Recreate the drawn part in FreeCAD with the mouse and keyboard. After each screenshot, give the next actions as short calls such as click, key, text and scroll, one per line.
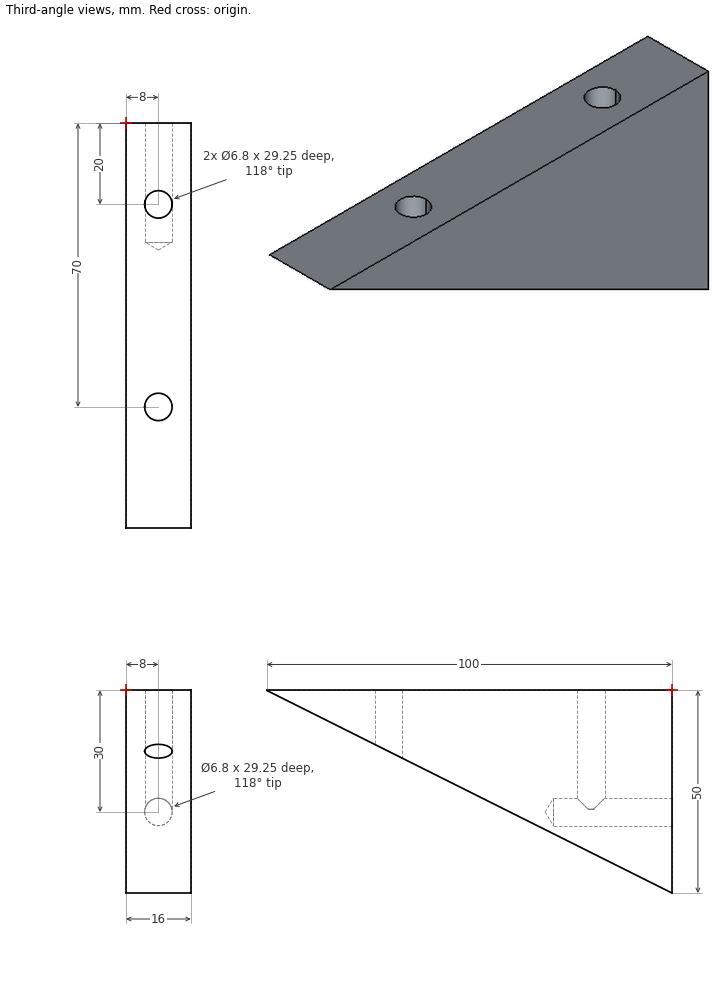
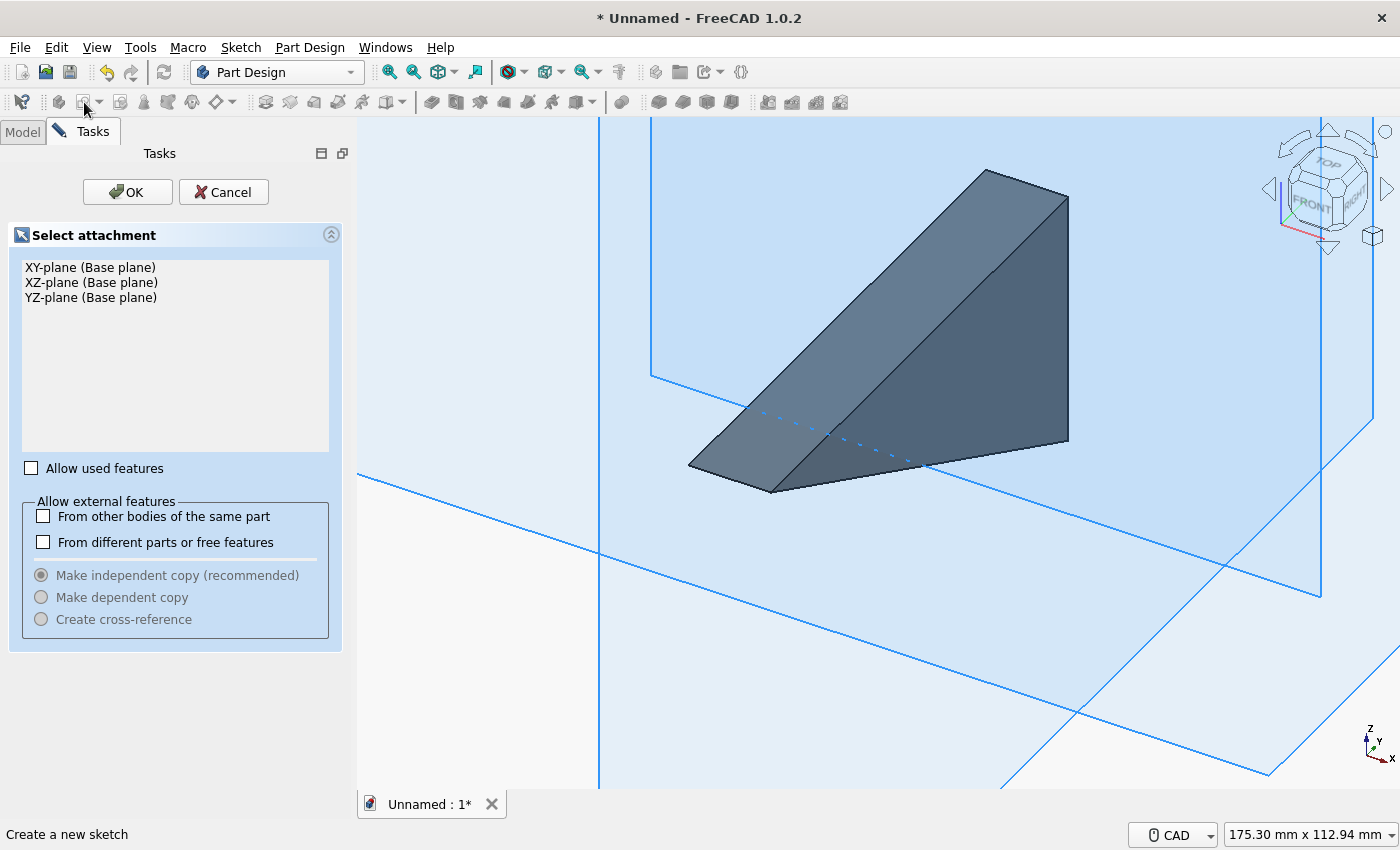
click(82, 282)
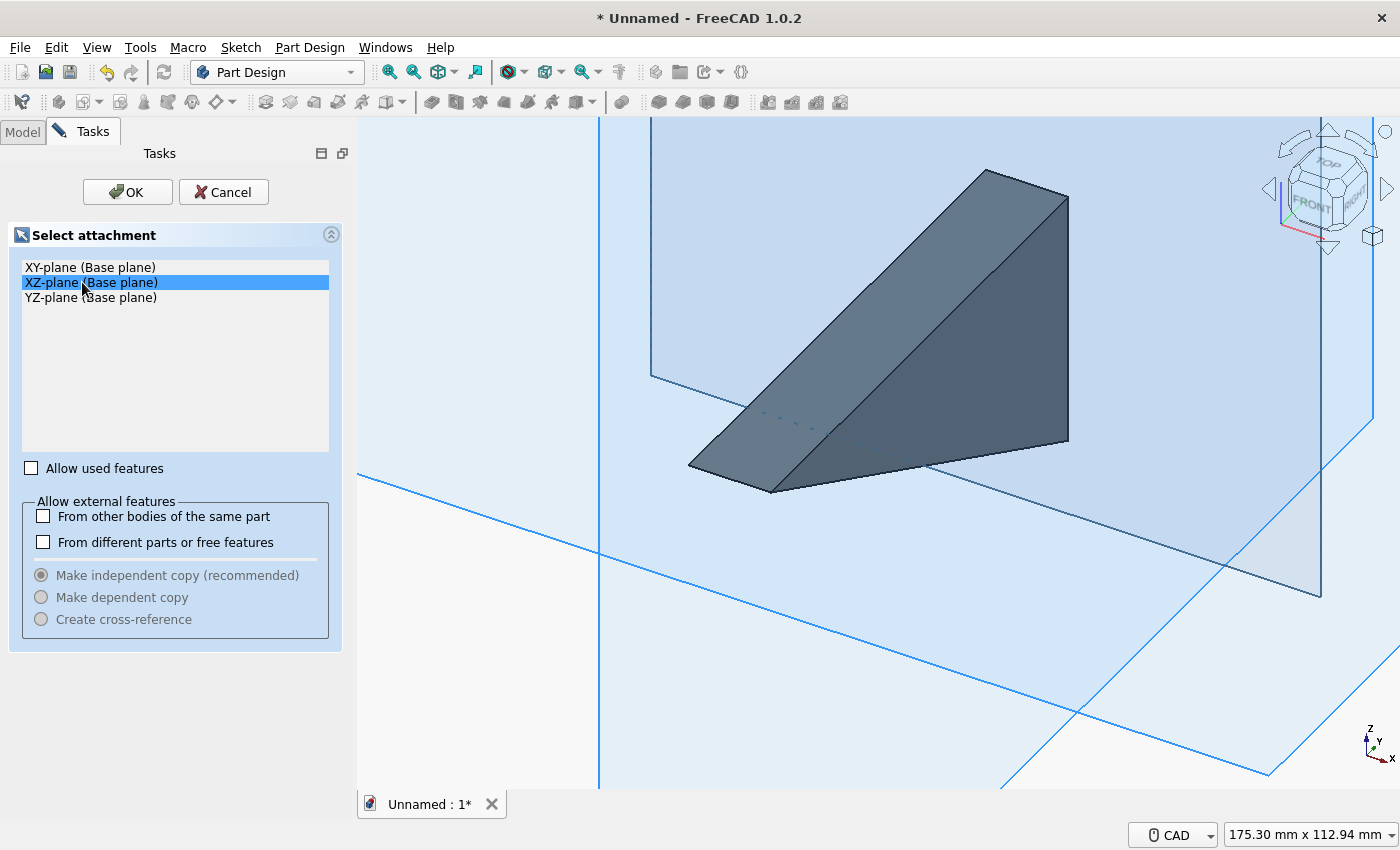
click(128, 192)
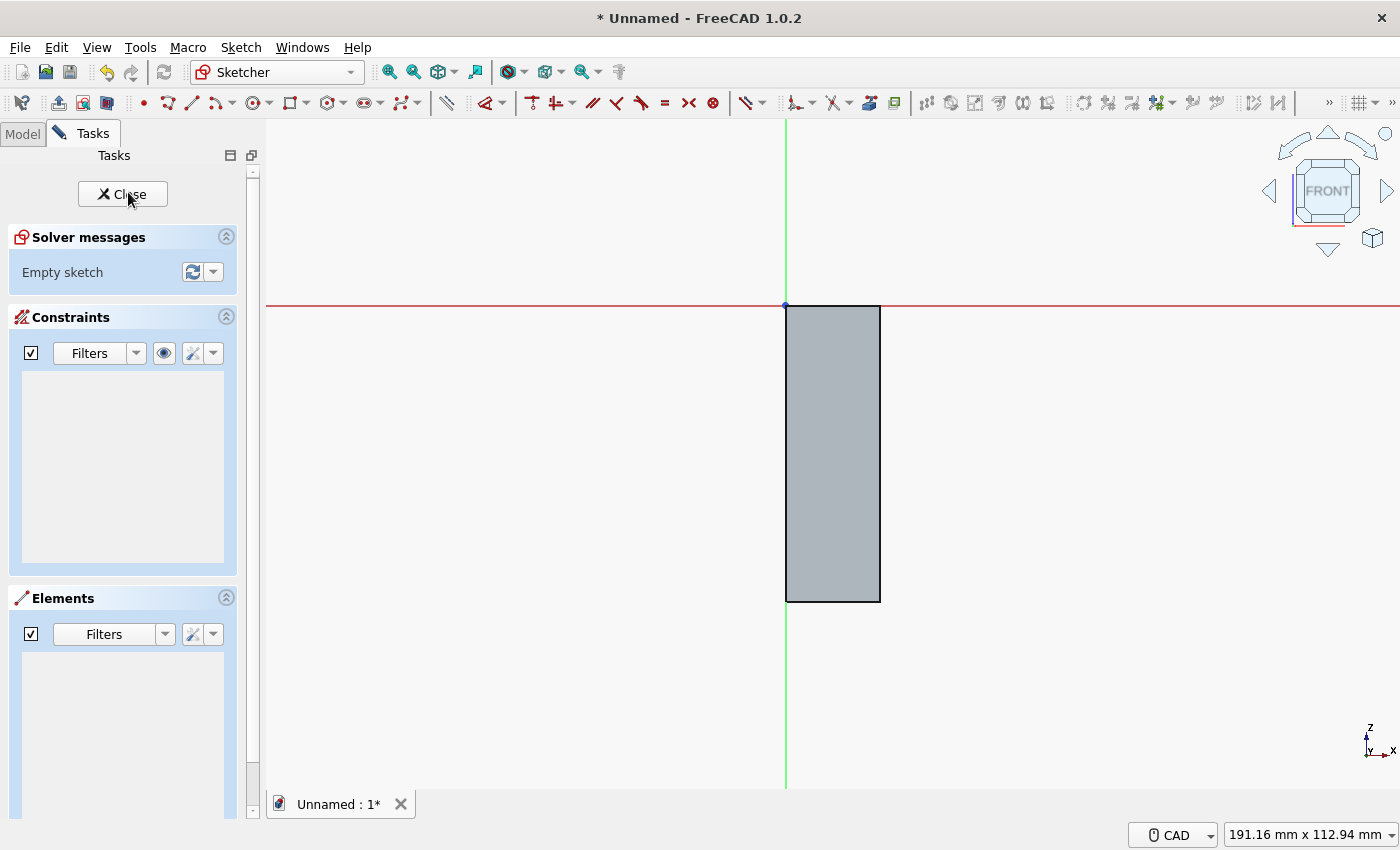
click(108, 104)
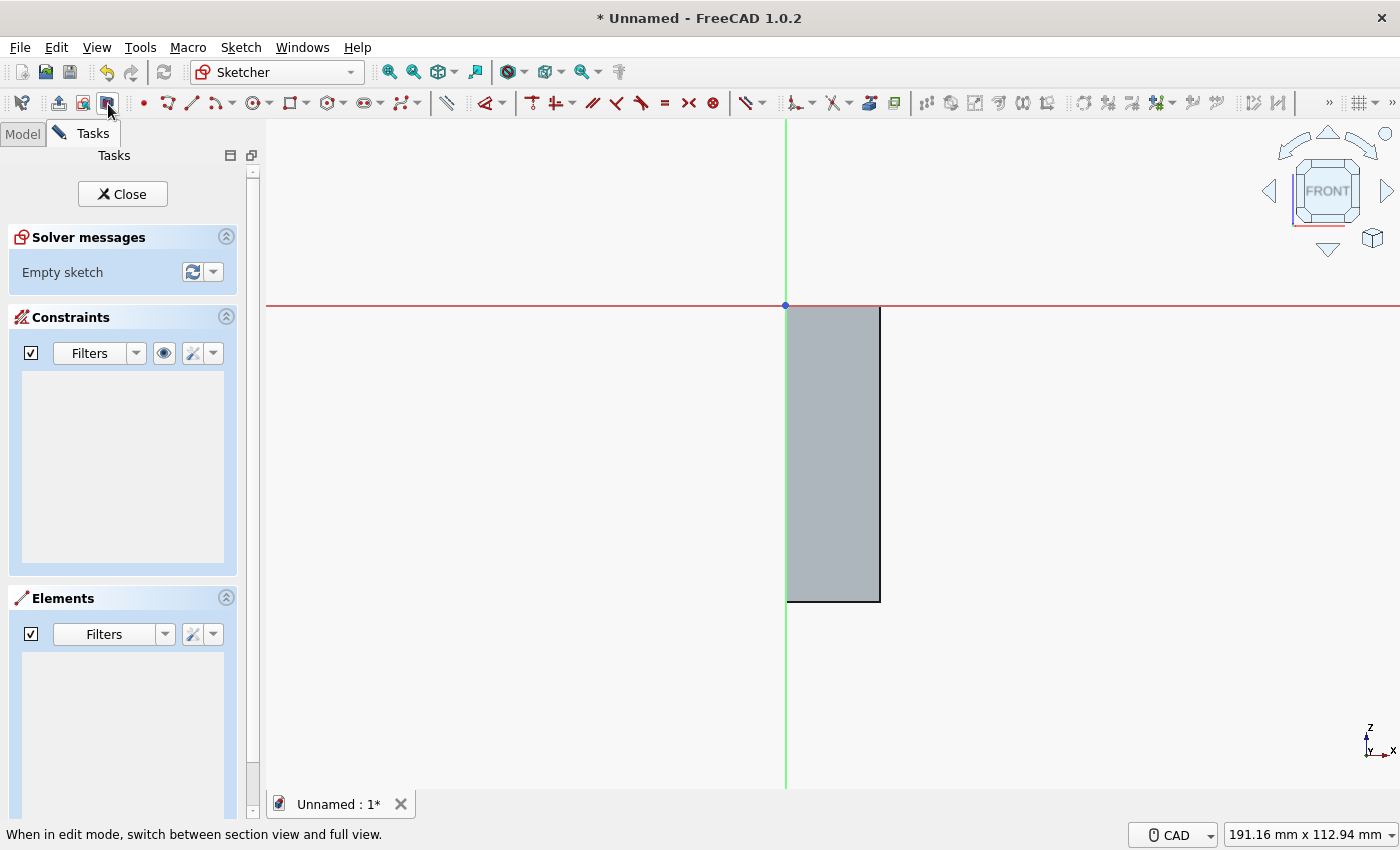
scroll(840, 487, up, 12)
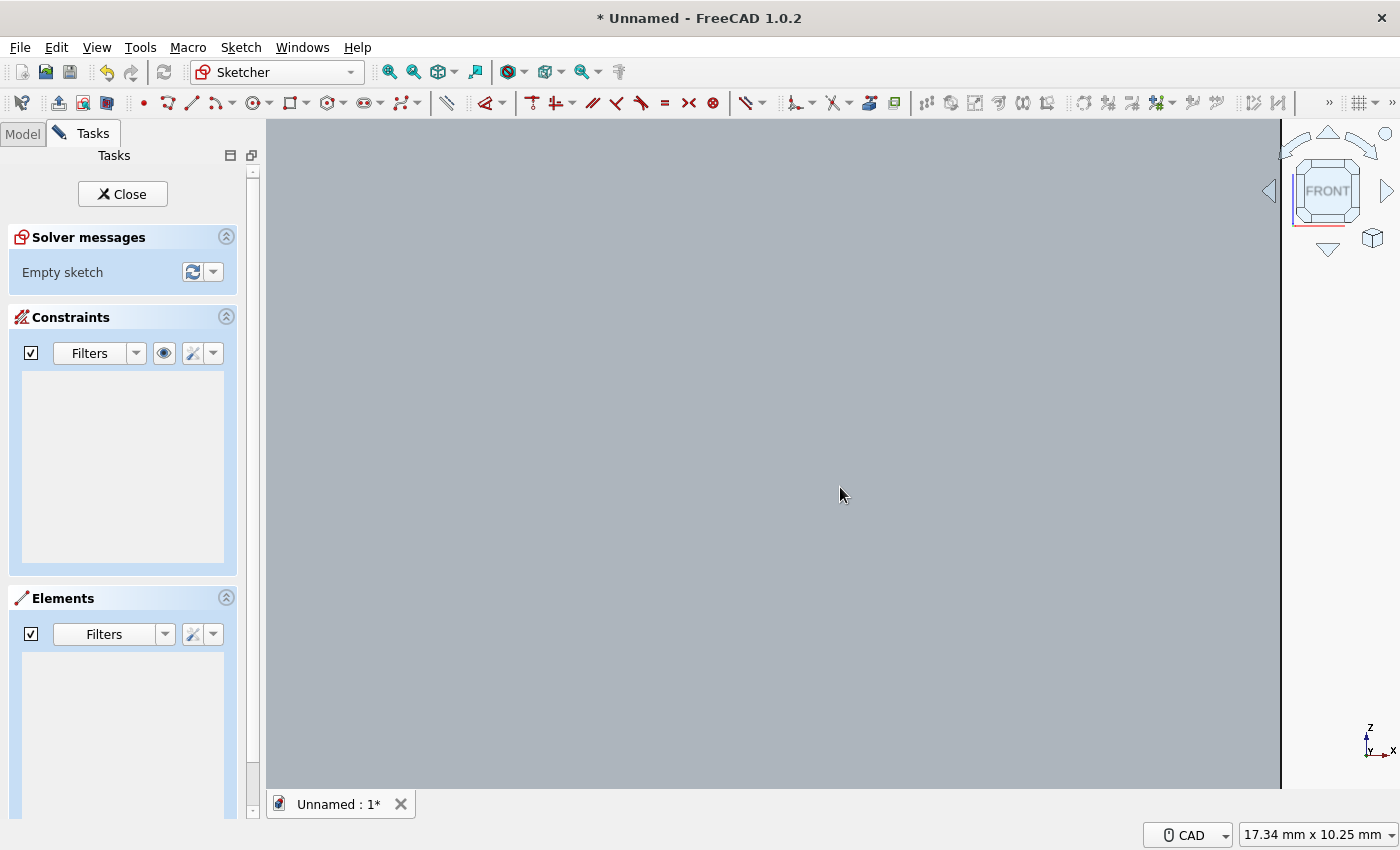
click(254, 104)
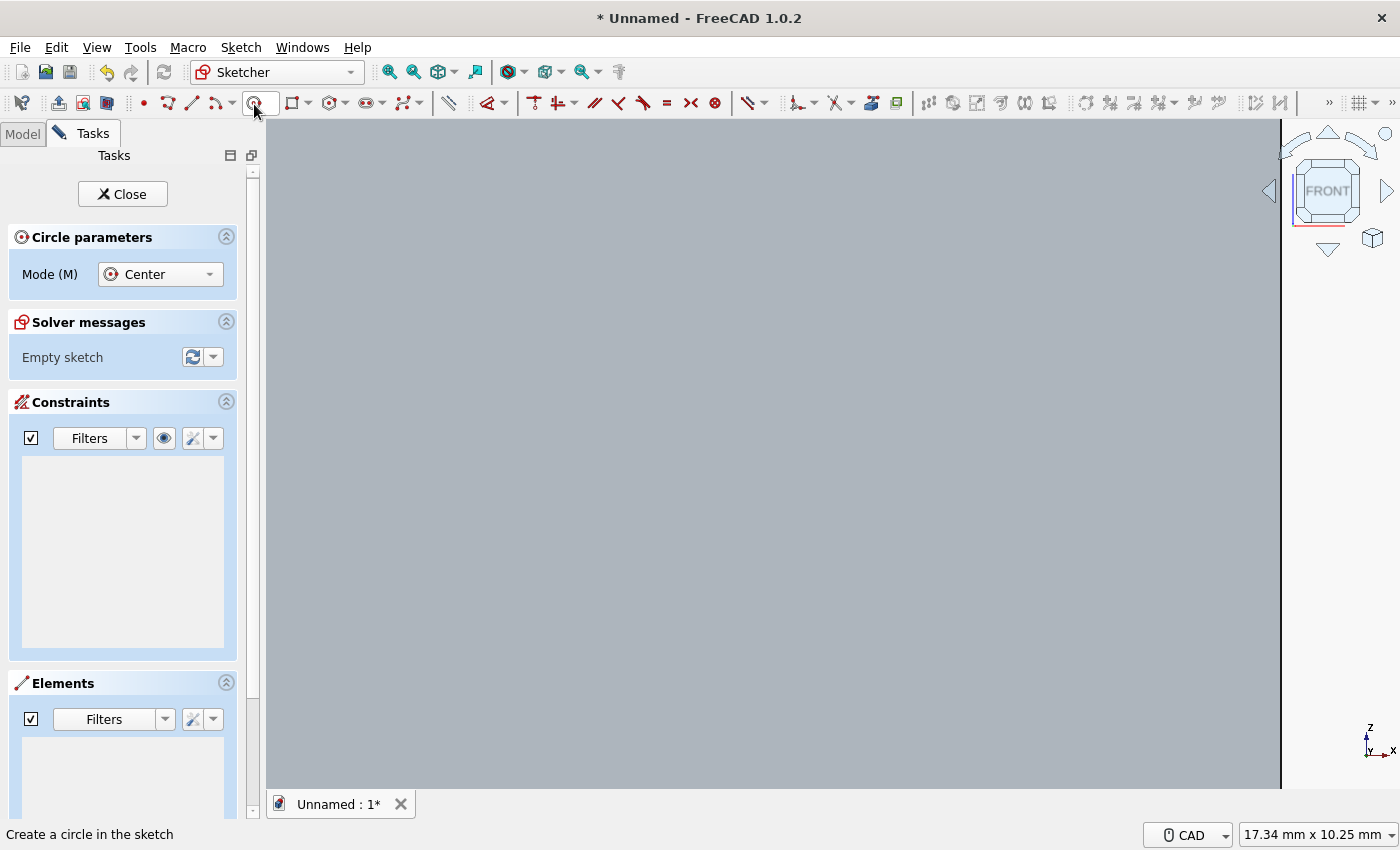
click(758, 445)
click(915, 287)
key(Escape)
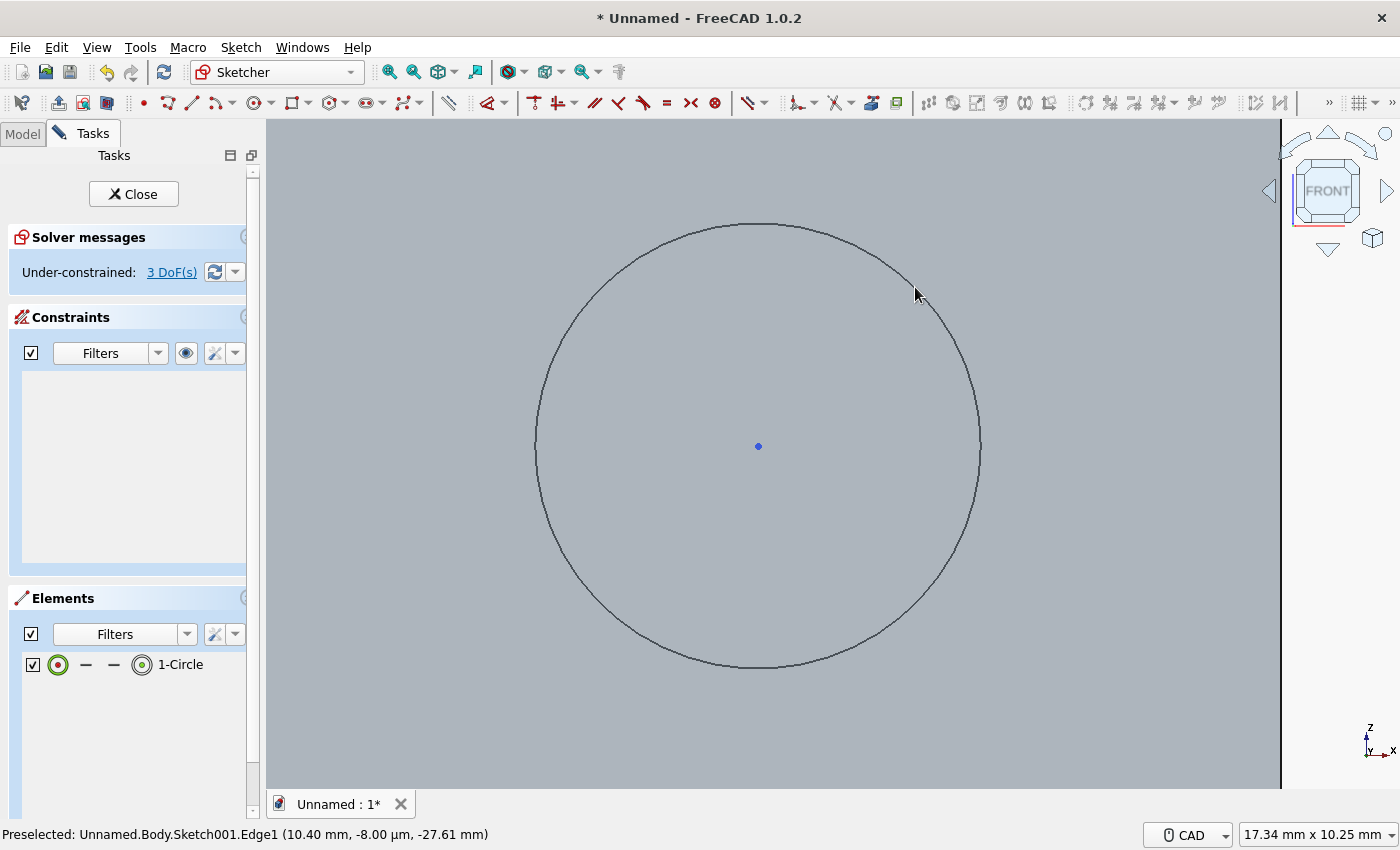
click(488, 104)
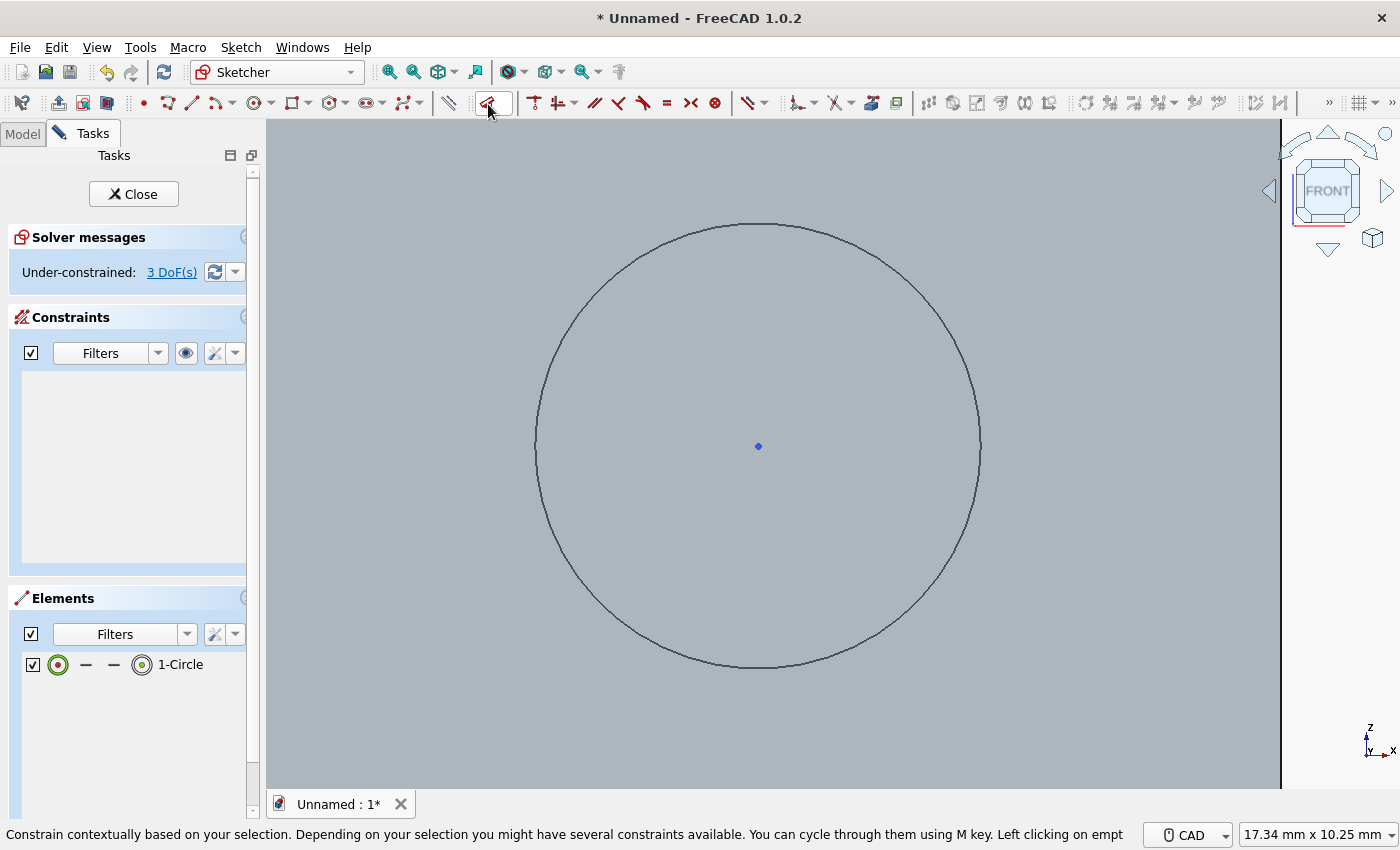
click(915, 288)
click(938, 265)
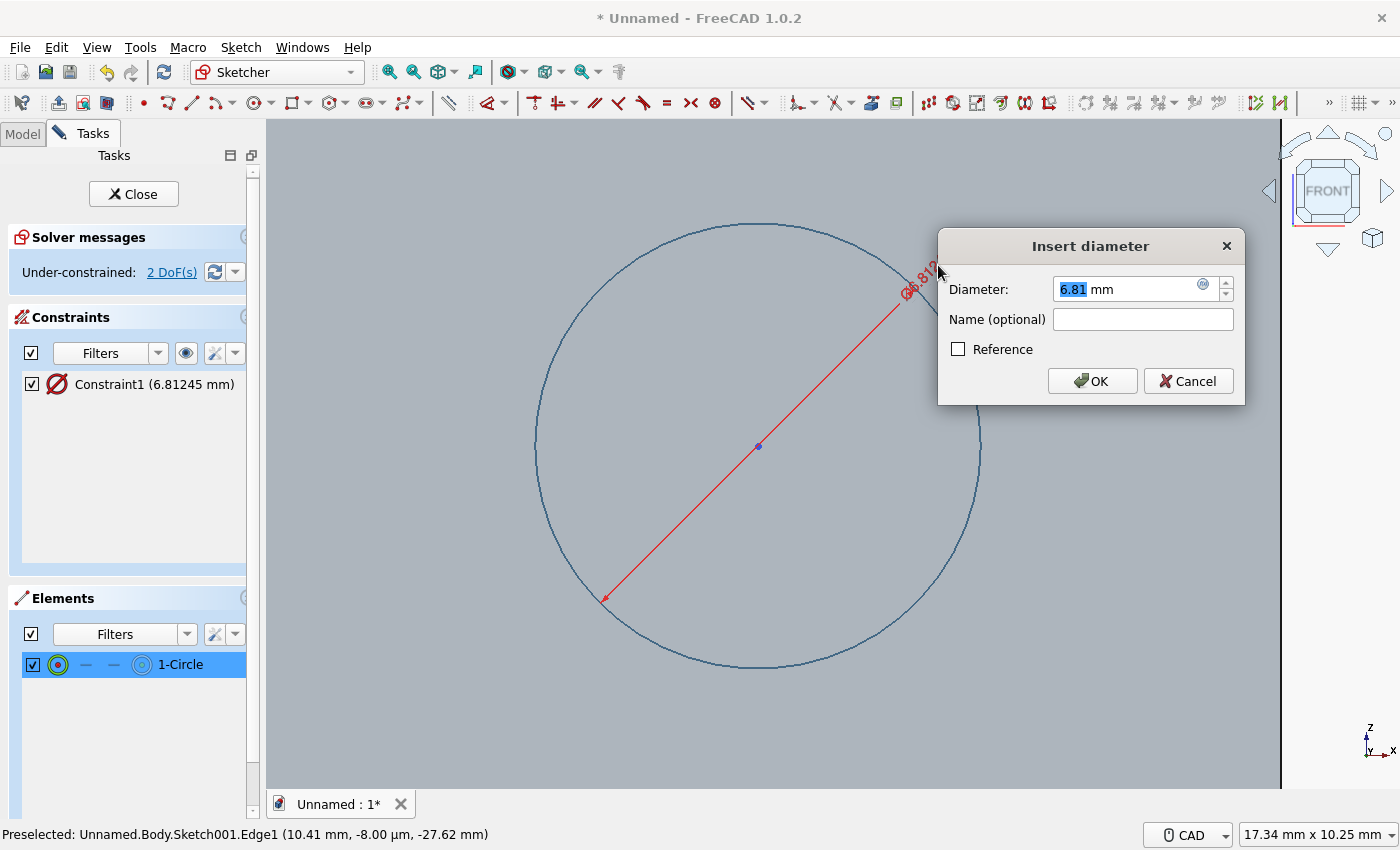
text(6.8)
key(Return)